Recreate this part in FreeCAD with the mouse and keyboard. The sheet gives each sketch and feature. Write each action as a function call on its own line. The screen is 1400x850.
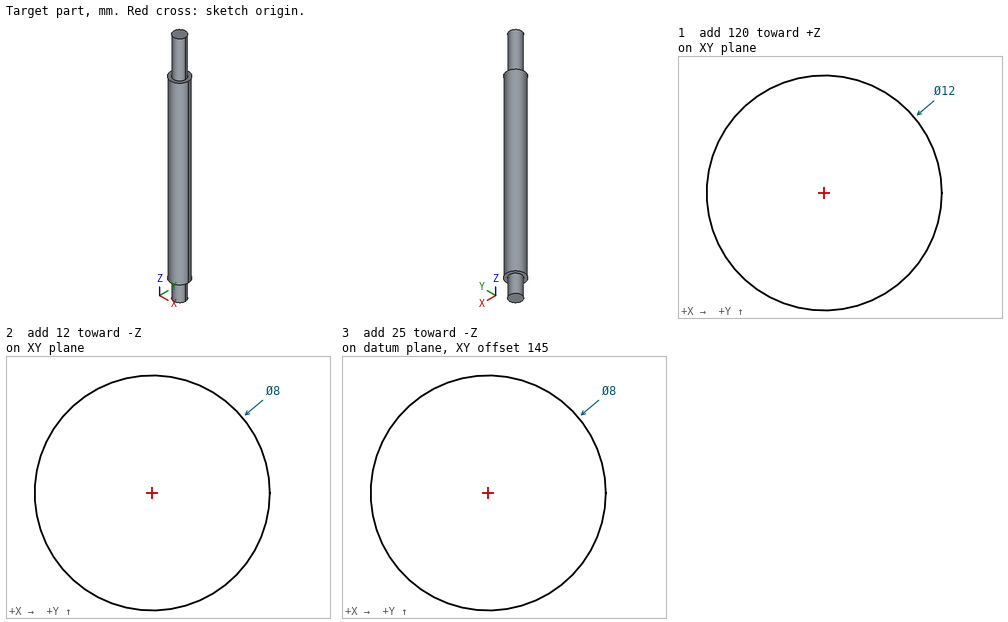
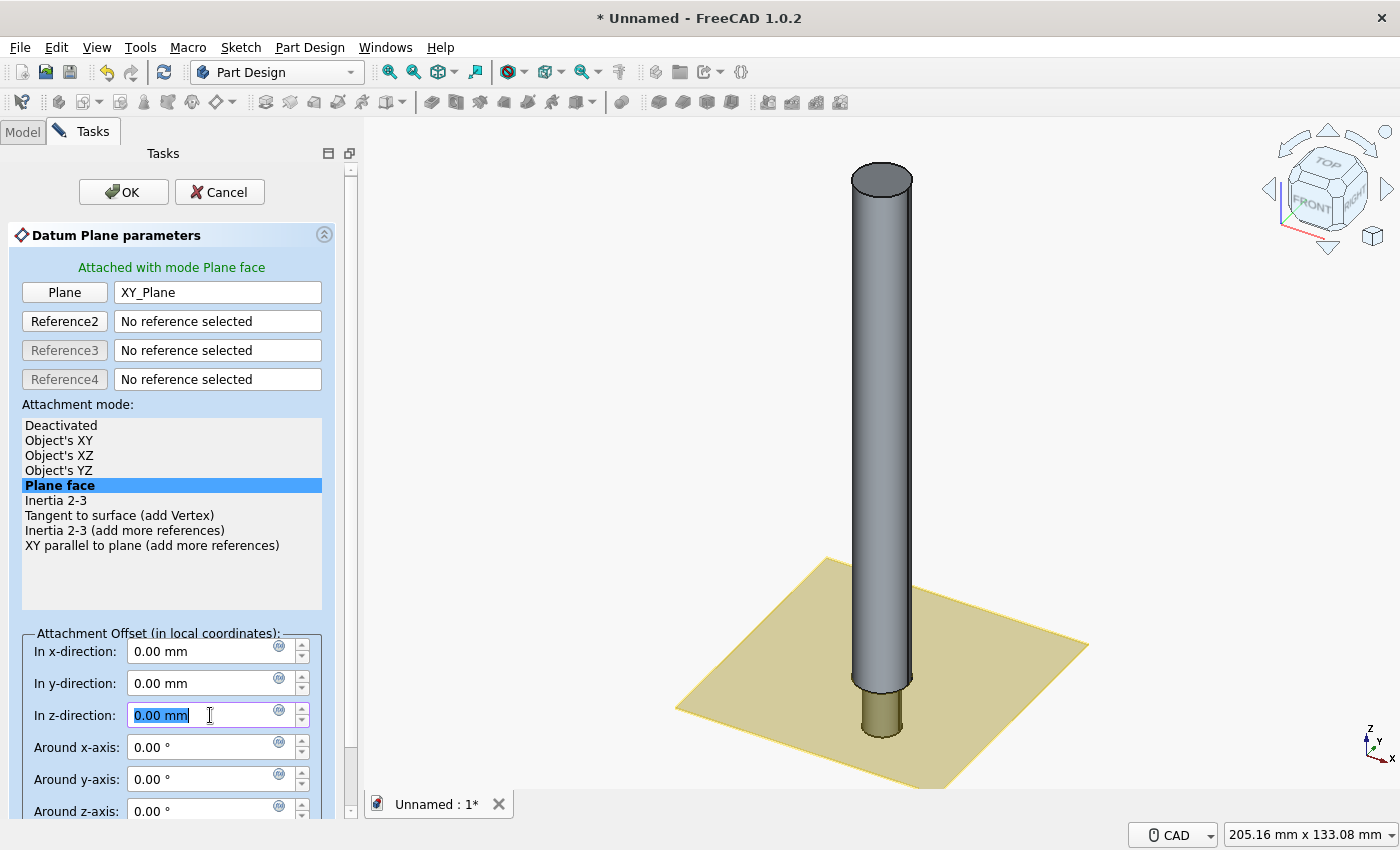
text(145)
key(Tab)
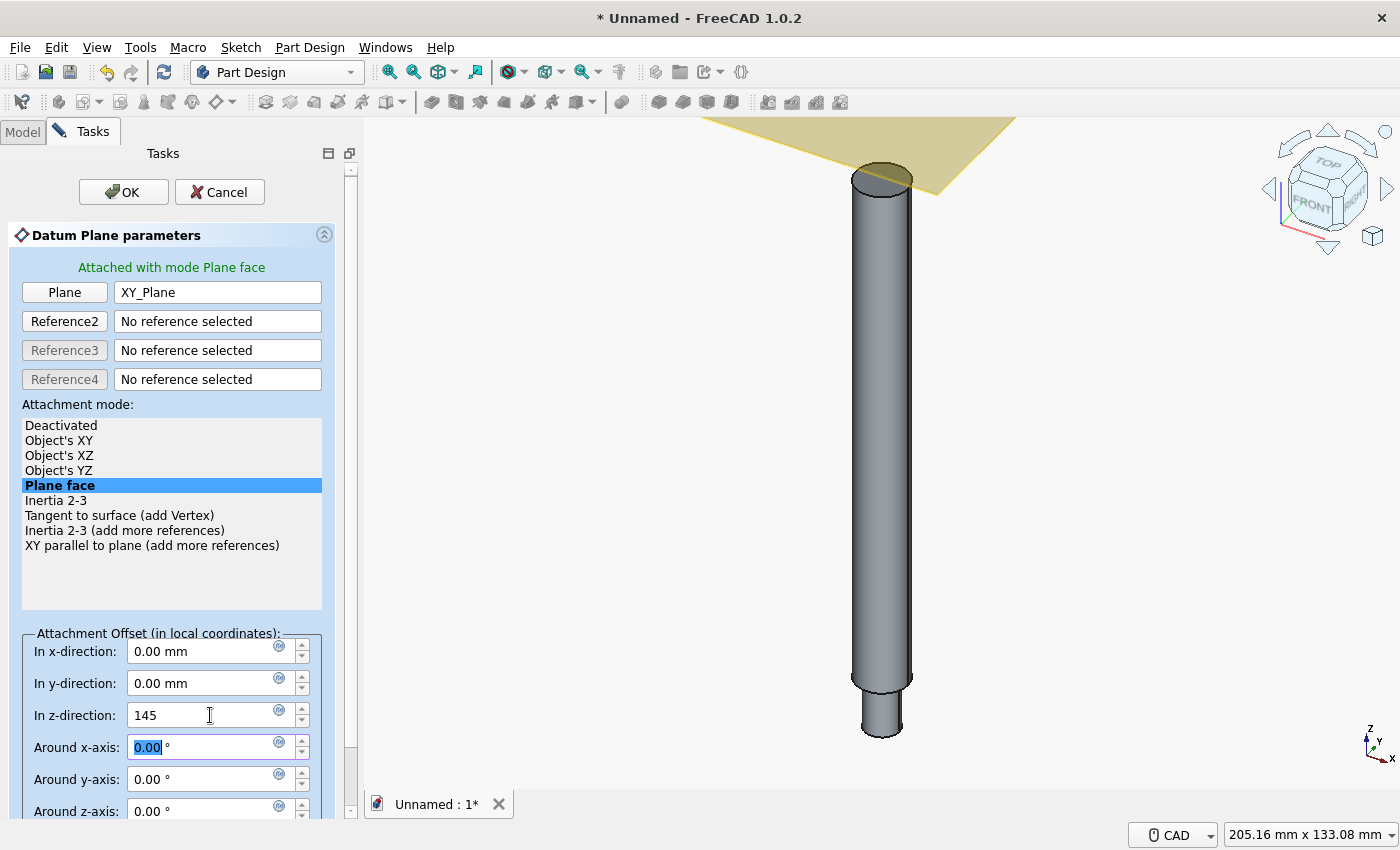
click(124, 192)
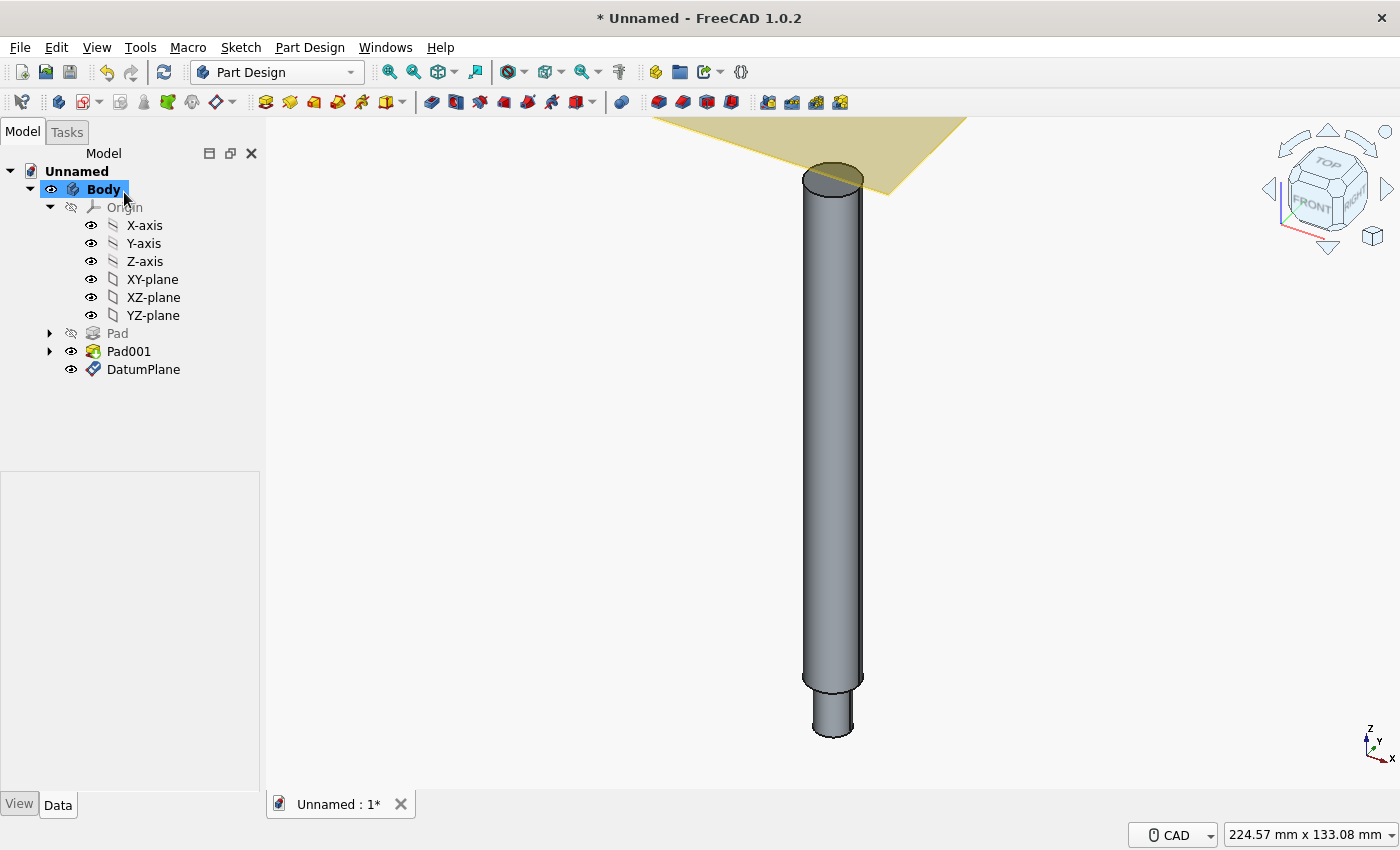
click(116, 369)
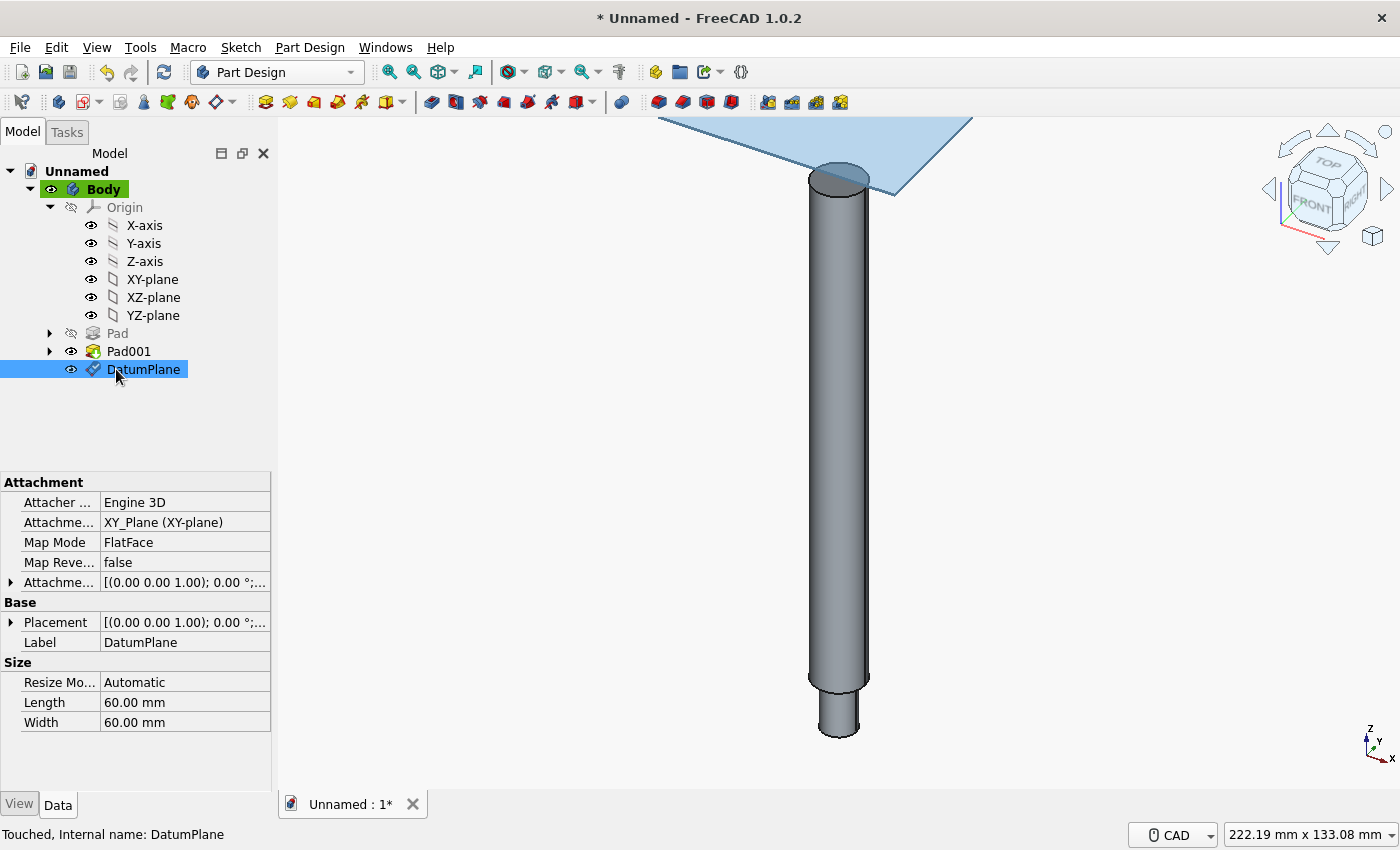
click(84, 102)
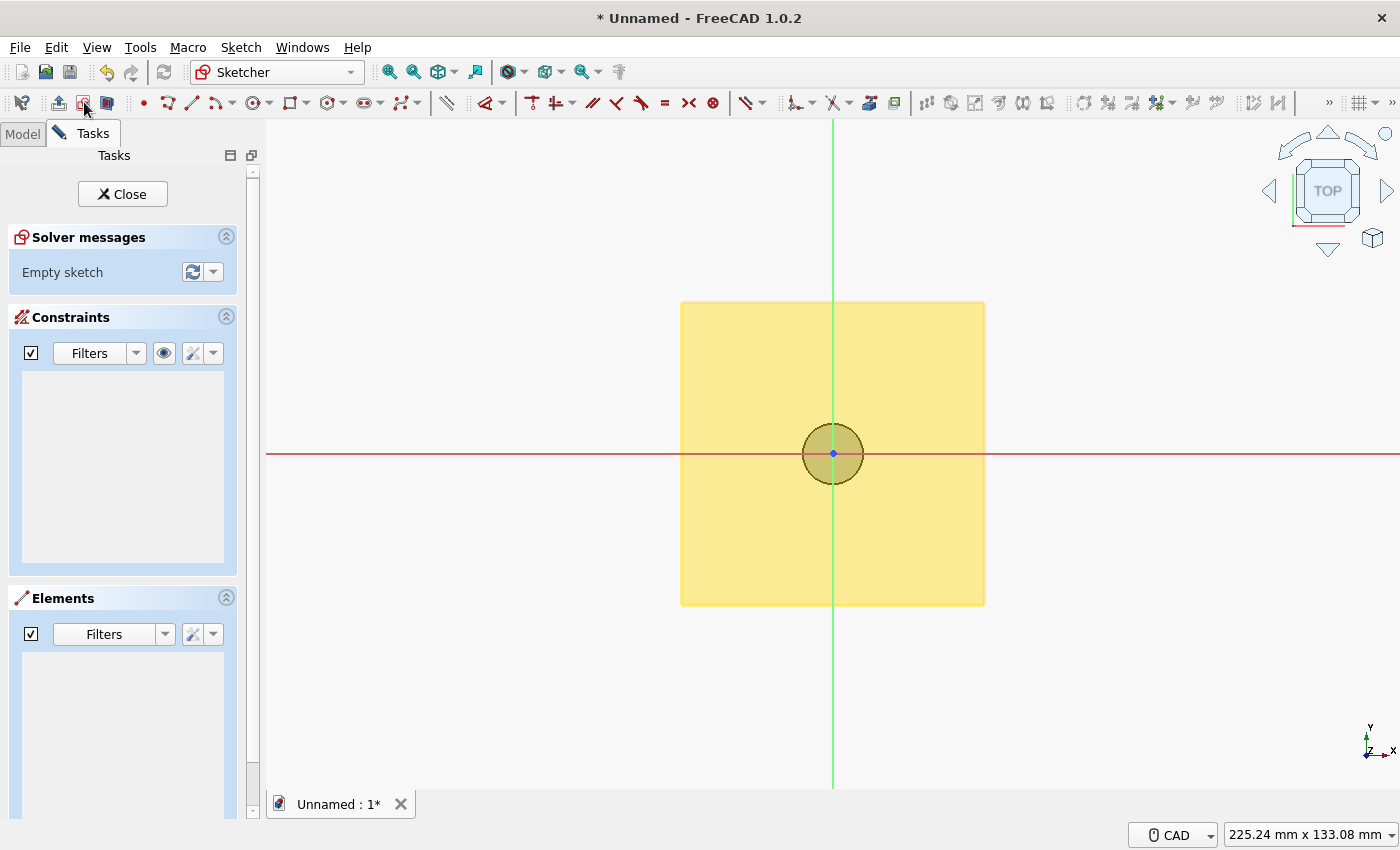
scroll(840, 454, up, 12)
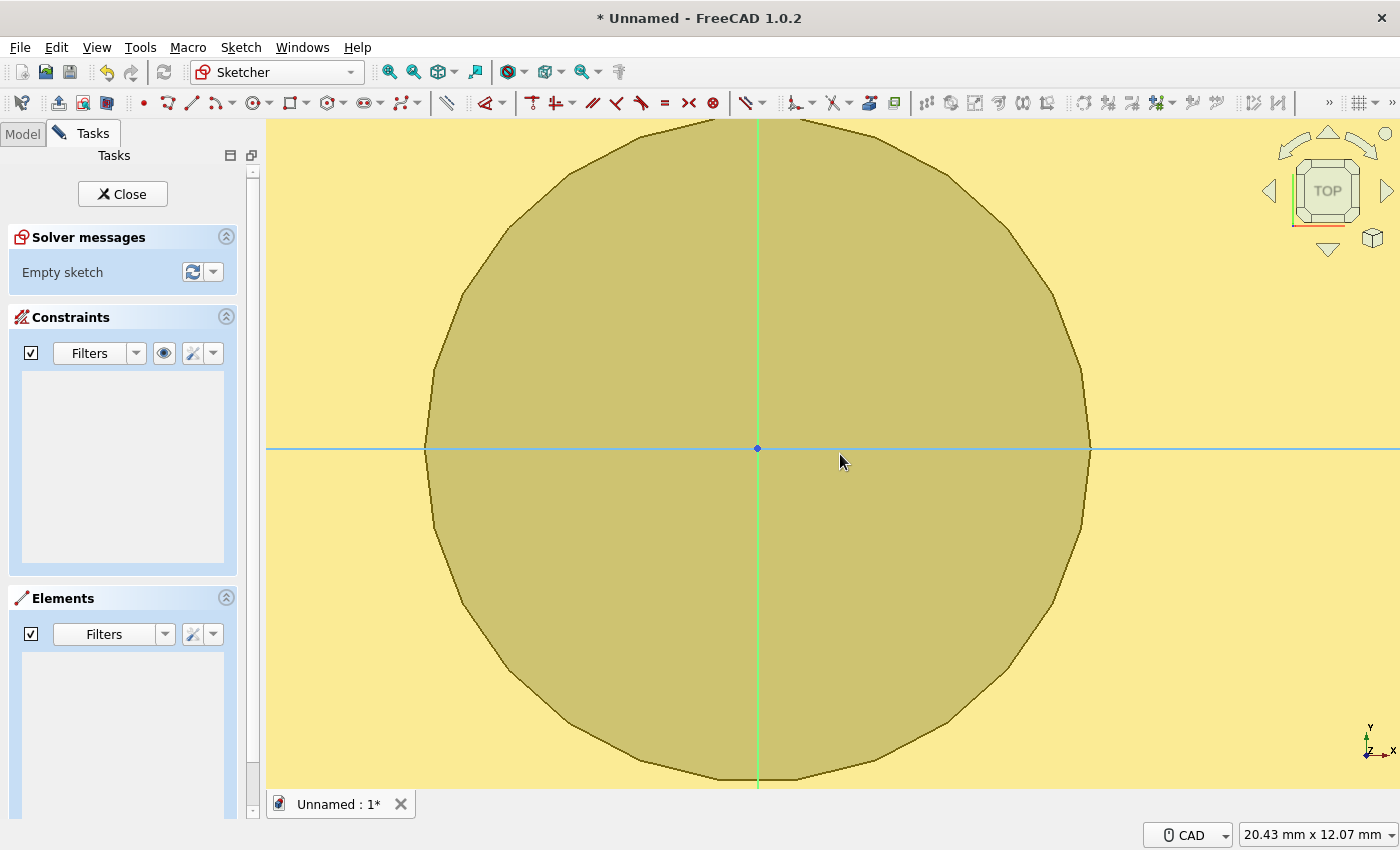
key(g)
key(c)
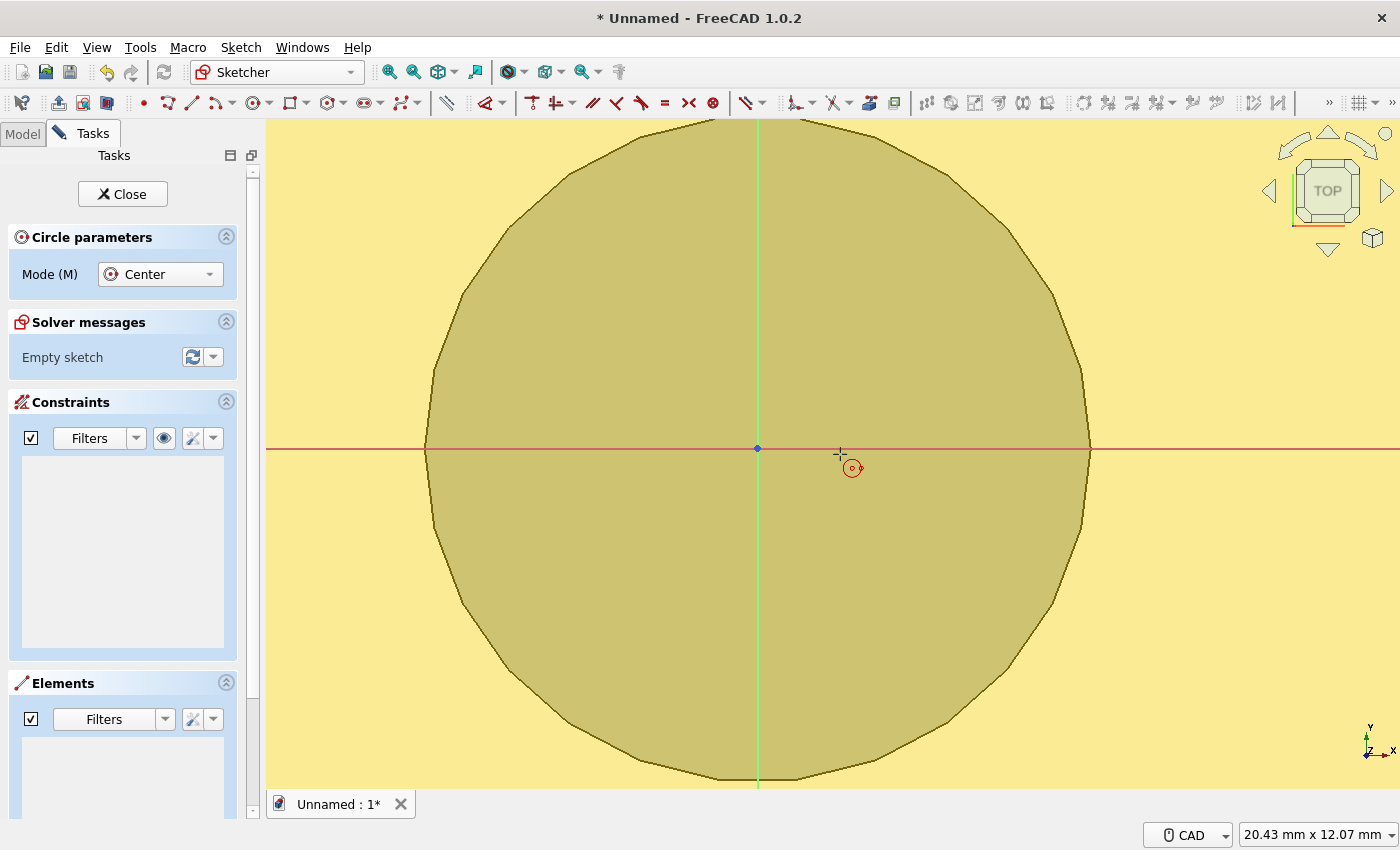
click(758, 449)
click(915, 292)
key(Escape)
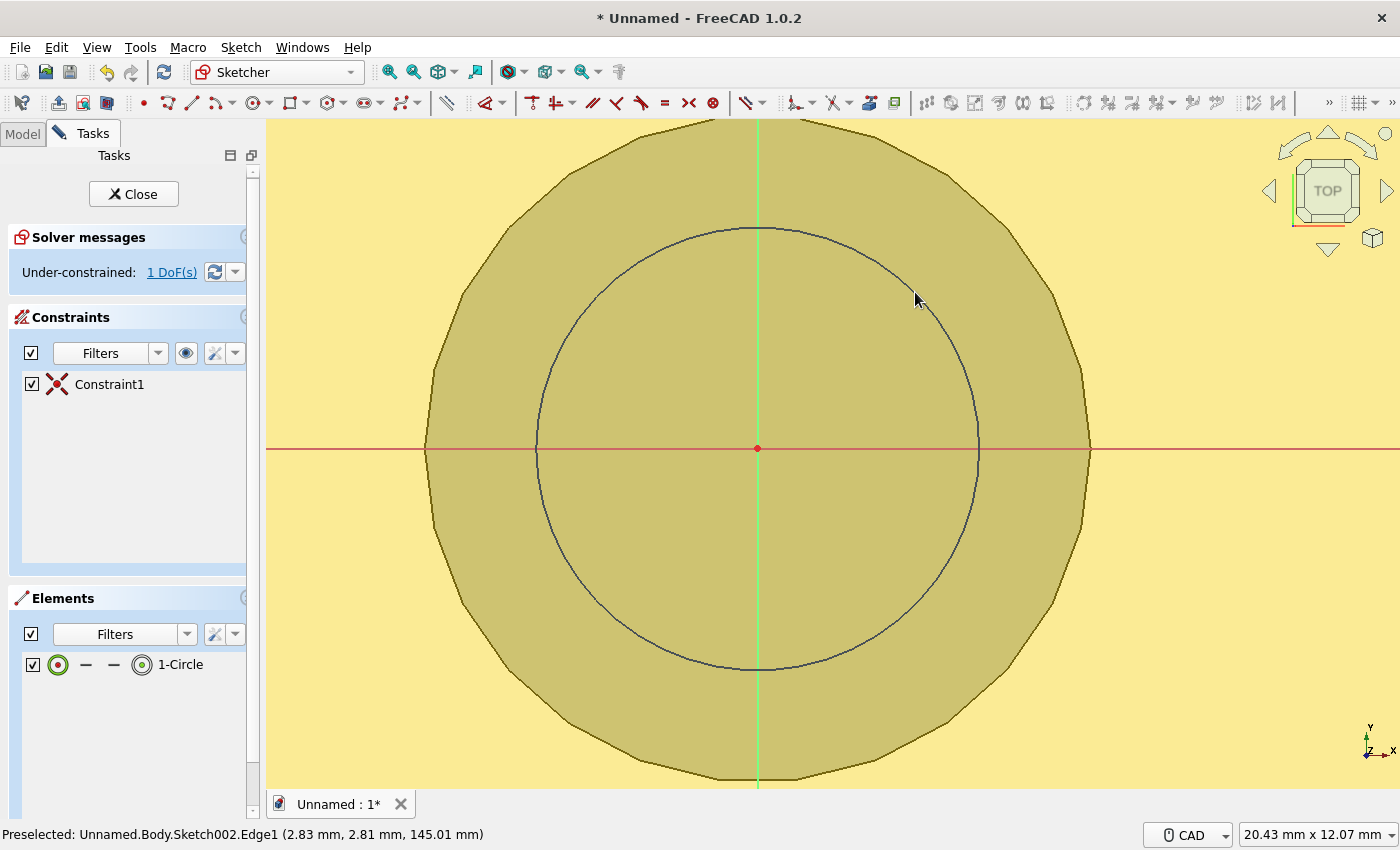
key(d)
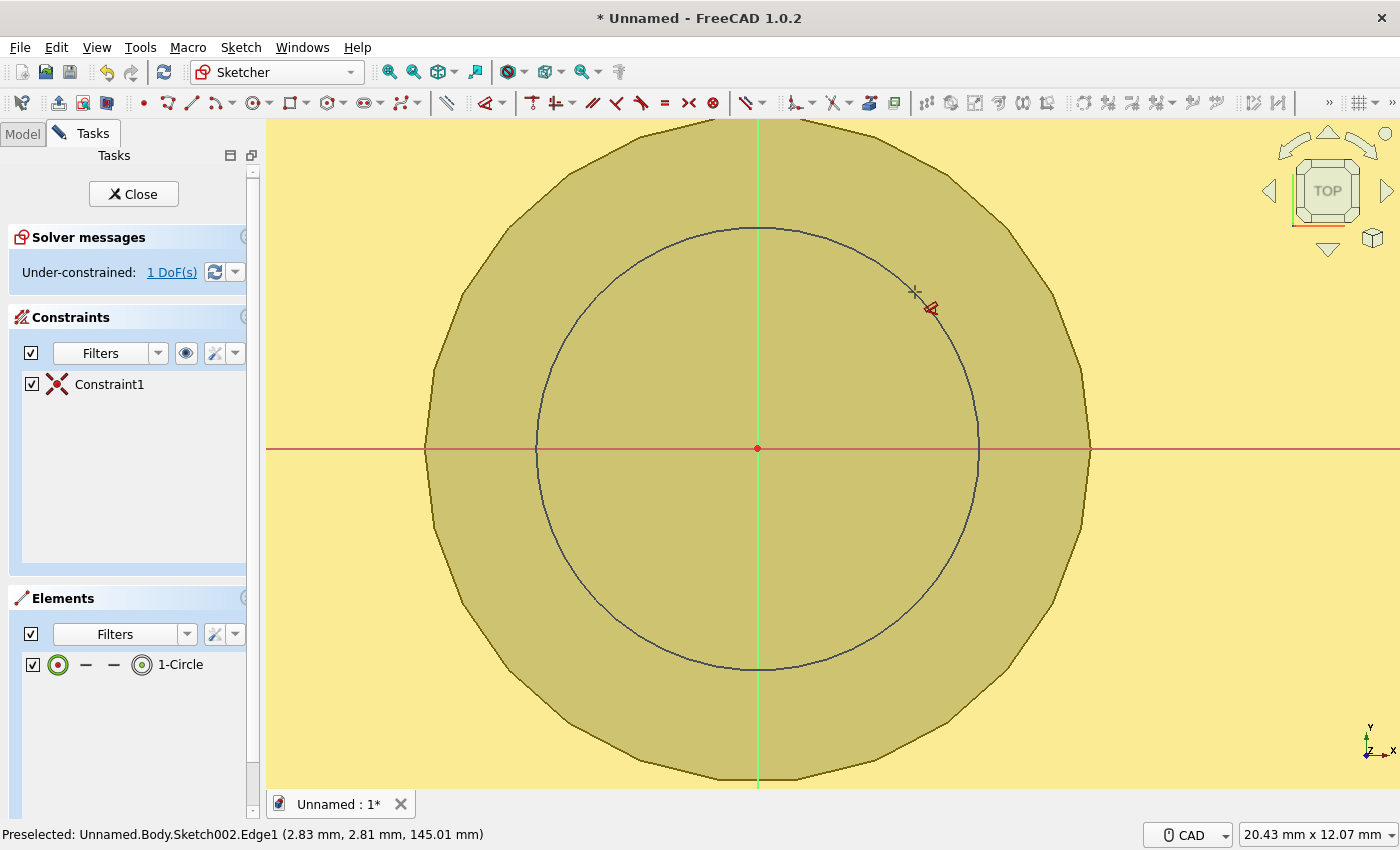
click(914, 292)
click(937, 269)